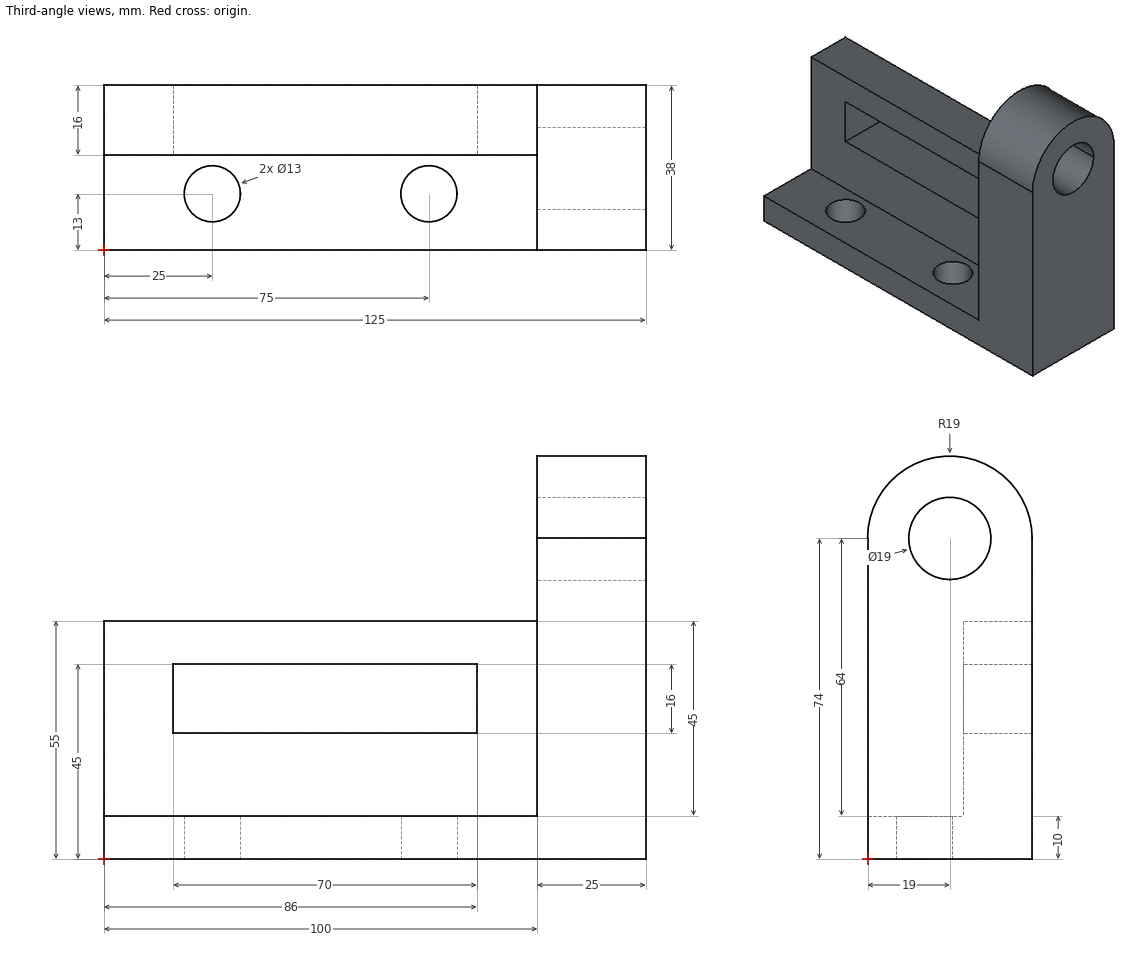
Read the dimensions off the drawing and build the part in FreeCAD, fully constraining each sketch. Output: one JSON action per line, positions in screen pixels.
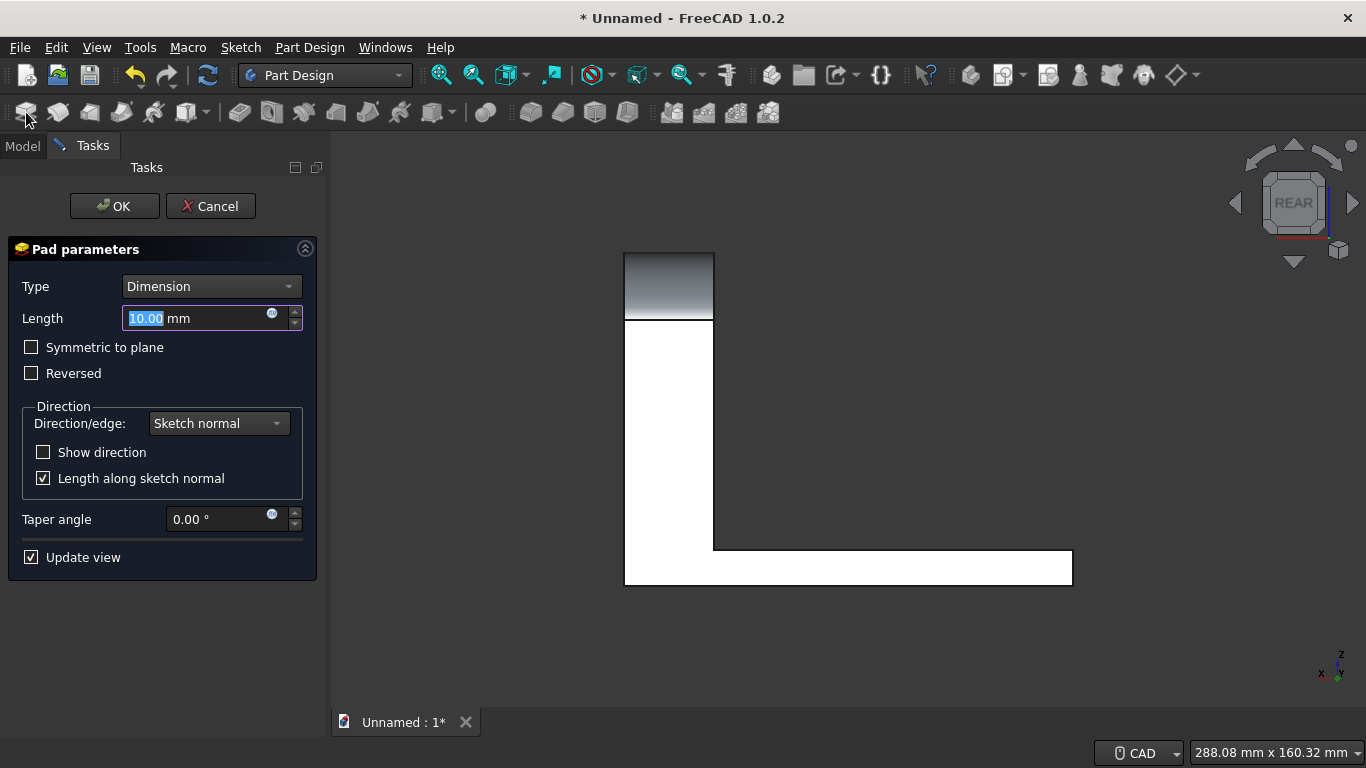
{"action": "type", "text": "16"}
{"action": "key", "text": "Tab"}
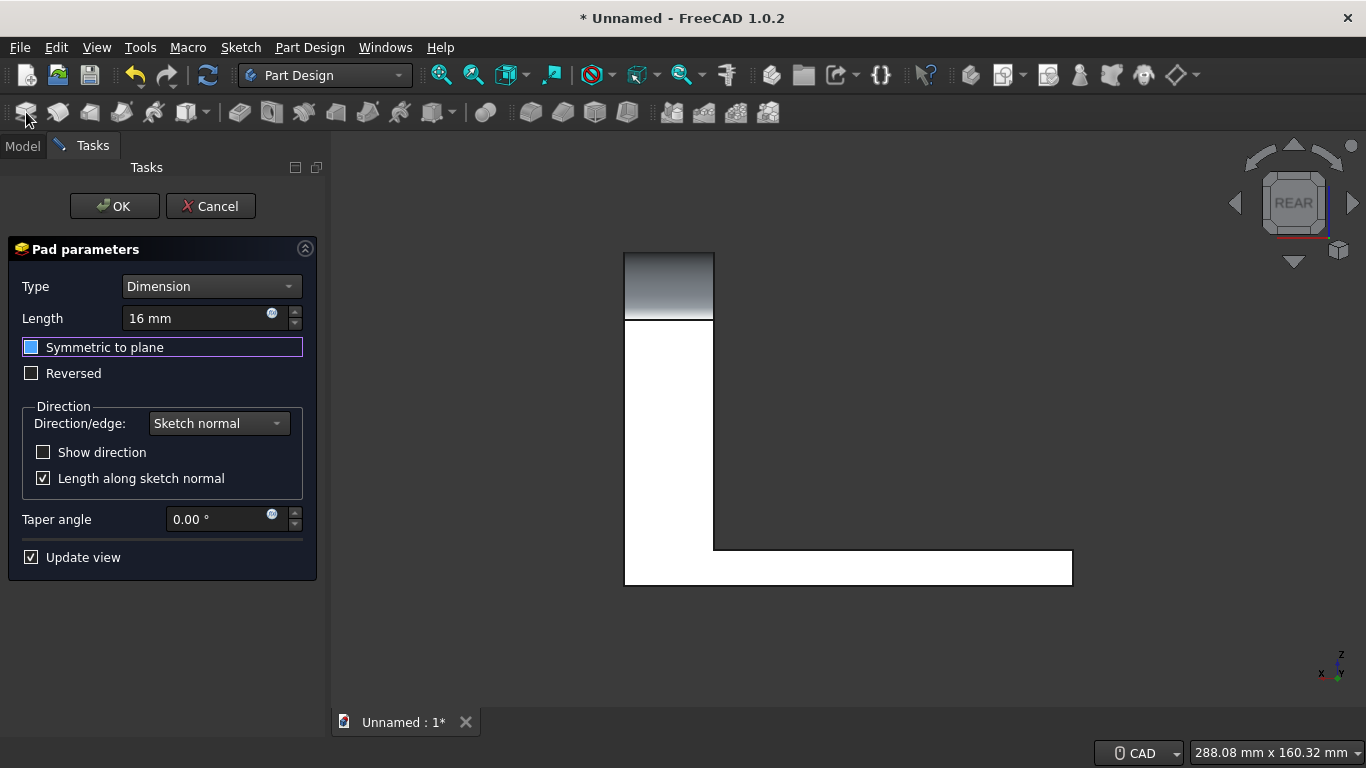
{"action": "left_click", "coordinate": [30, 373]}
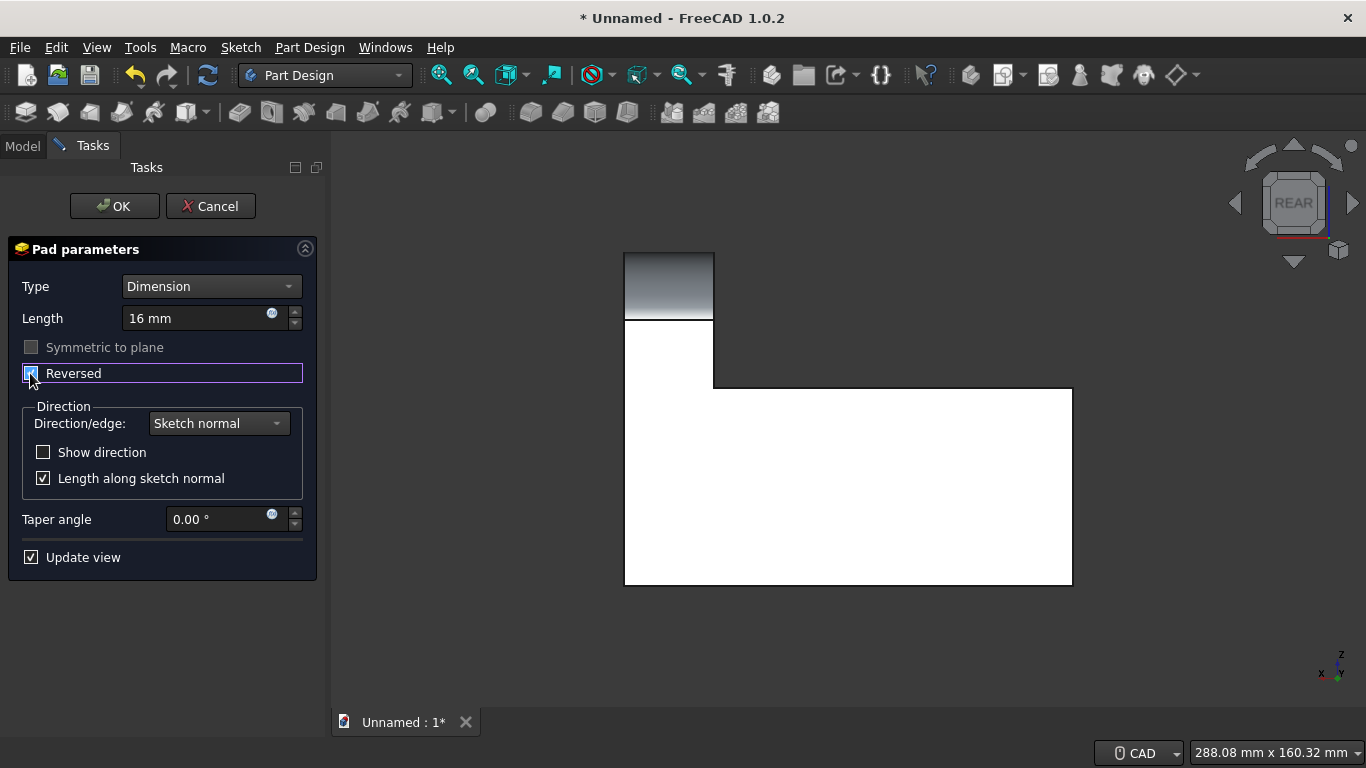
{"action": "left_click", "coordinate": [115, 206]}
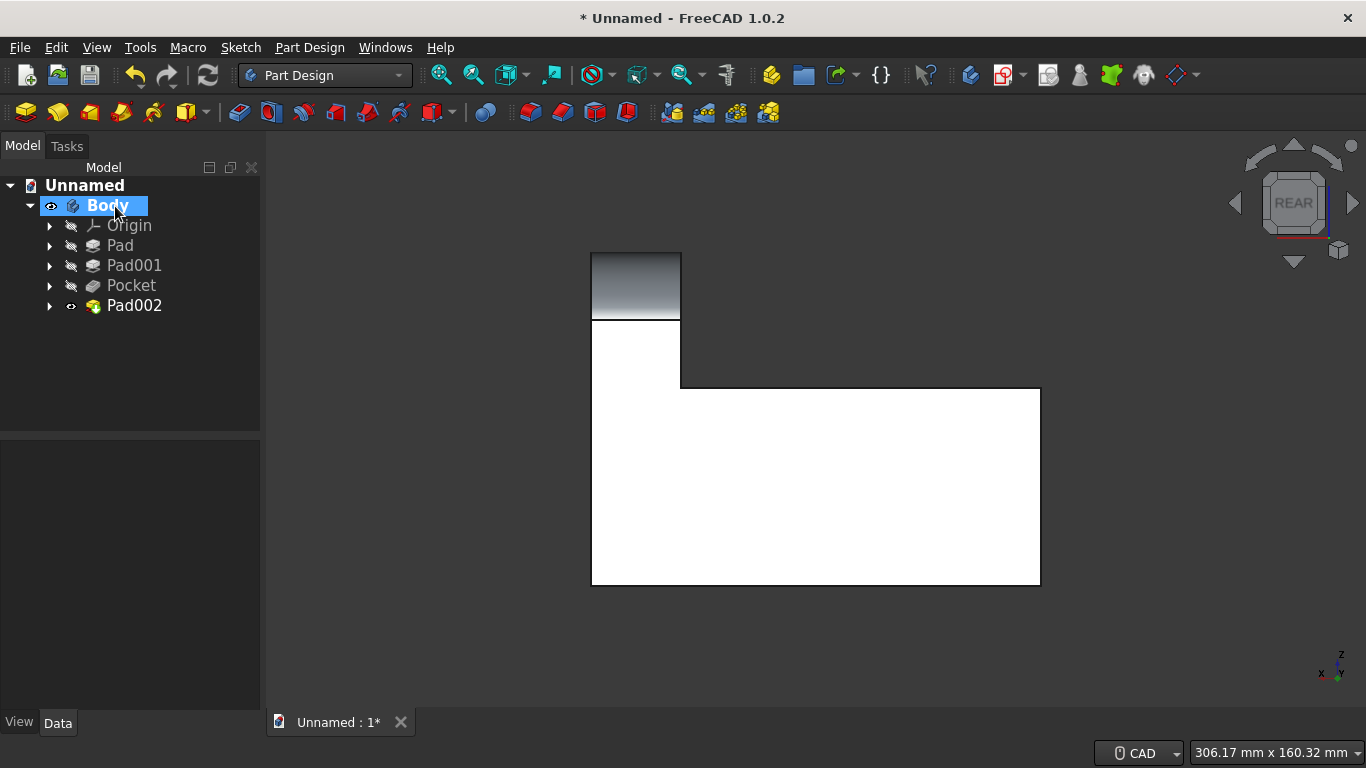
{"action": "left_click", "coordinate": [688, 490]}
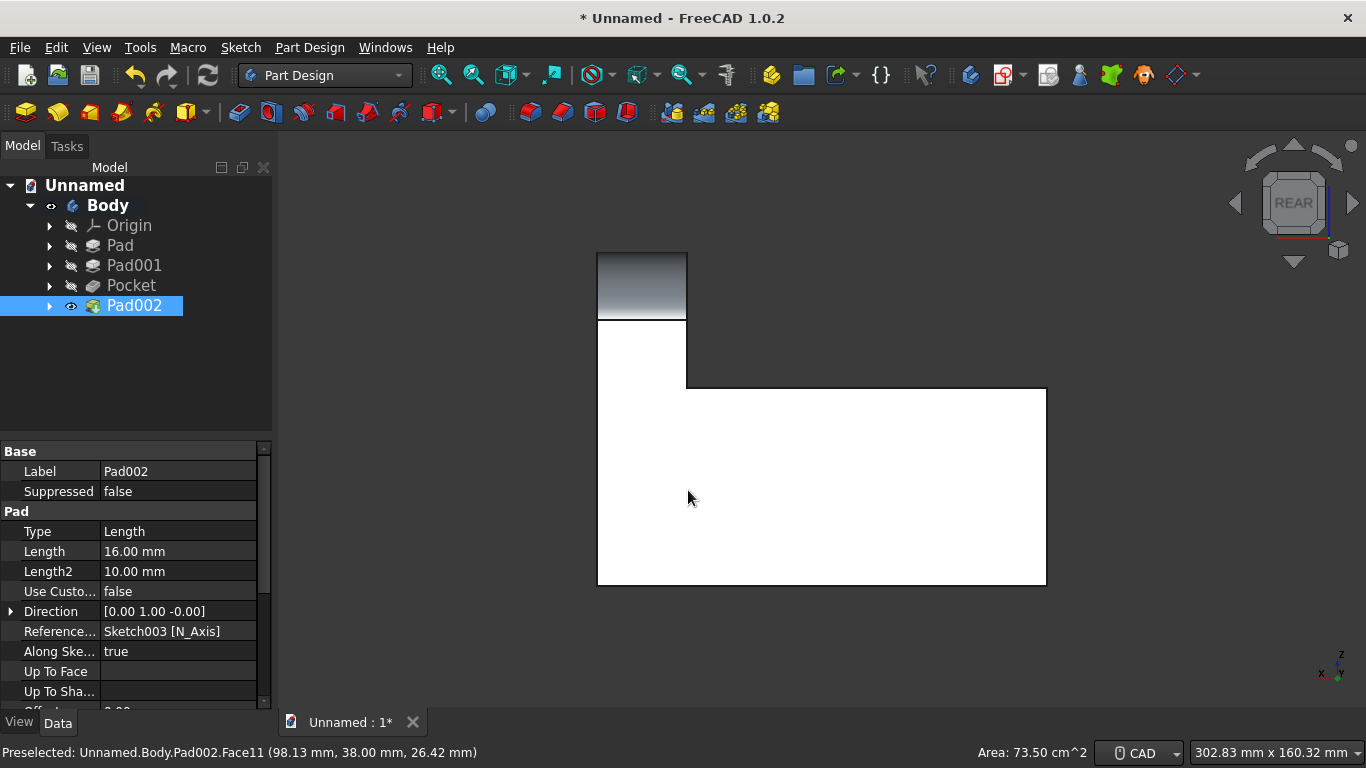
{"action": "left_click", "coordinate": [1004, 76]}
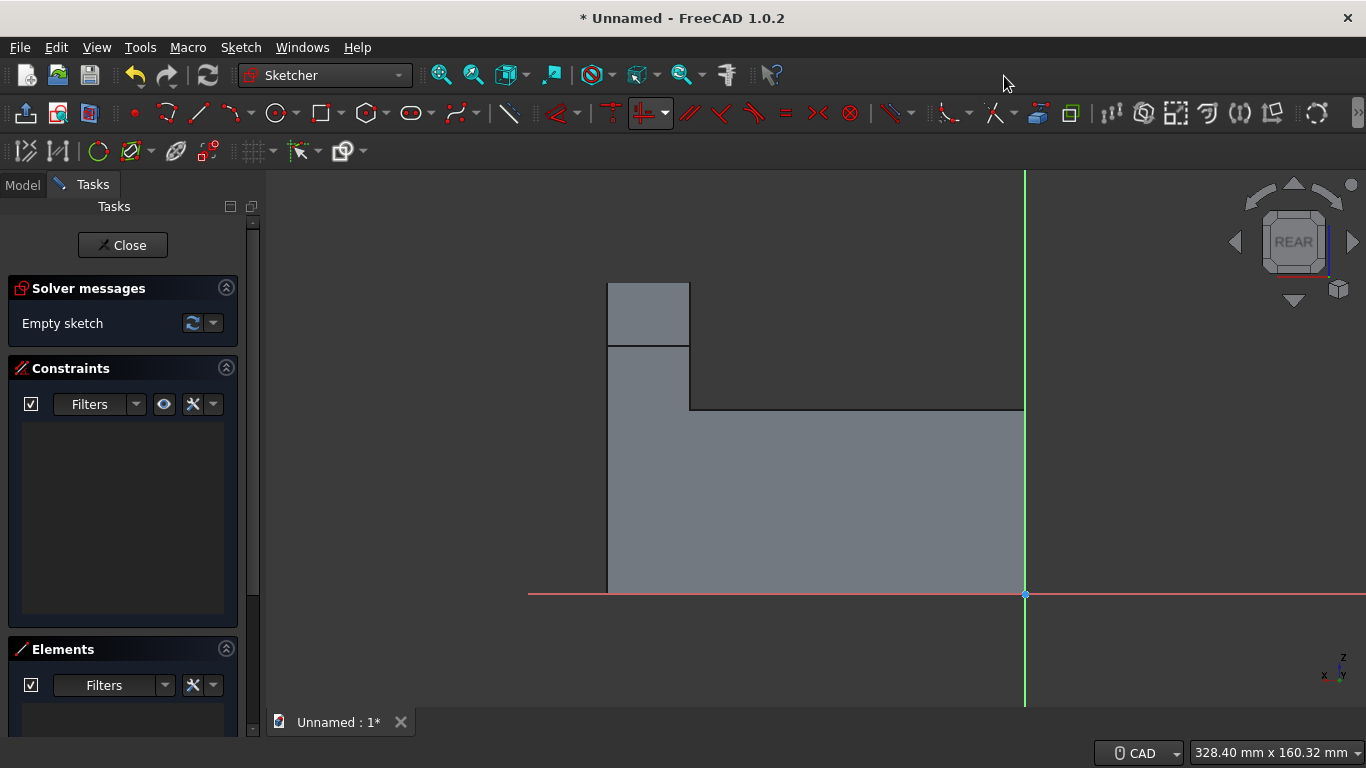
{"action": "scroll", "coordinate": [991, 584], "scroll_direction": "up", "scroll_amount": 4}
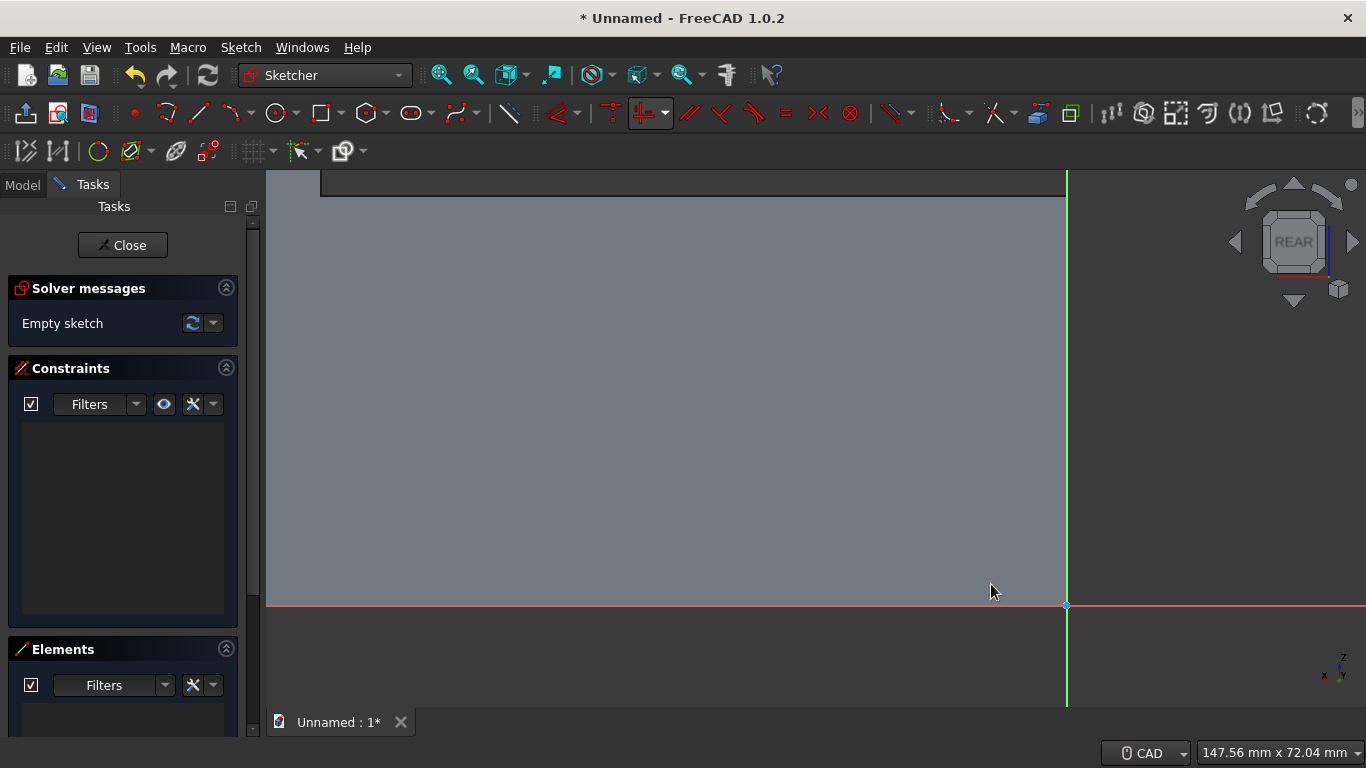
{"action": "left_click", "coordinate": [322, 114]}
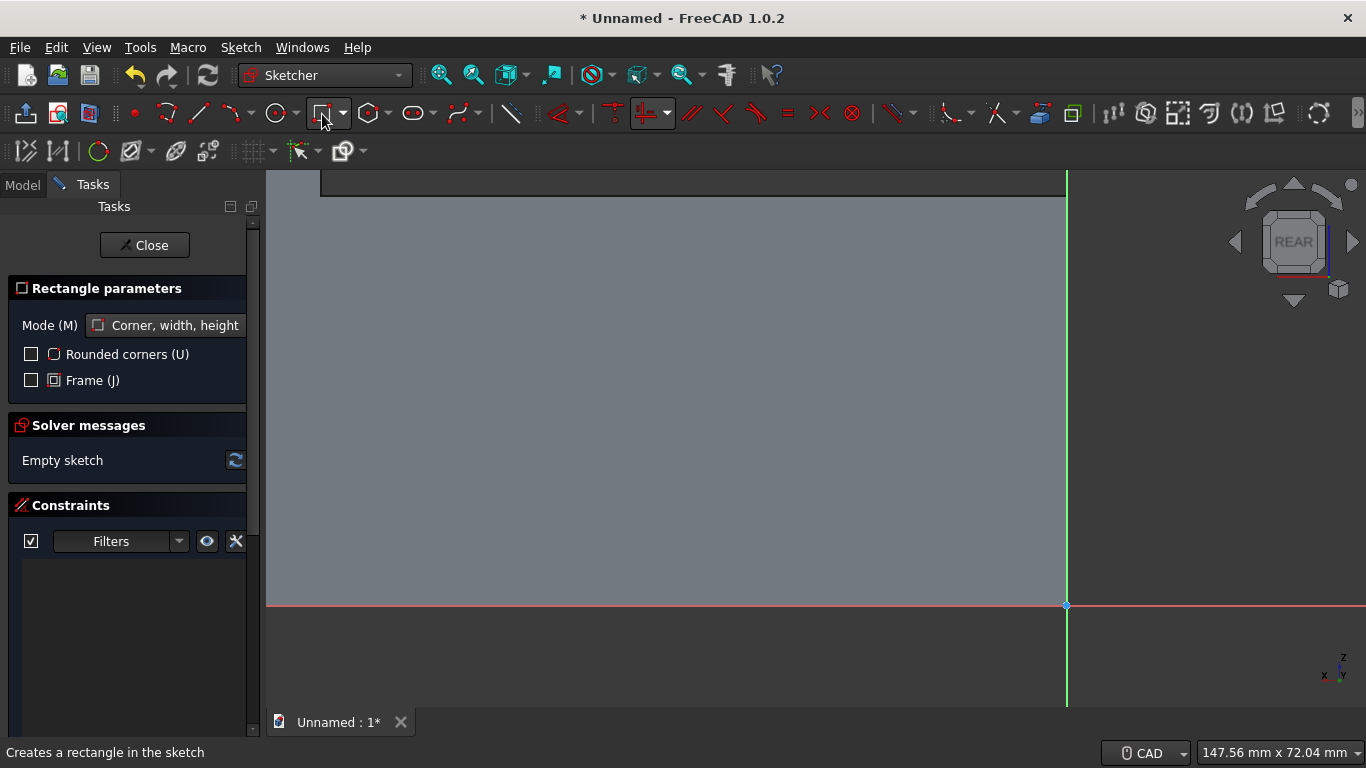
{"action": "left_click", "coordinate": [426, 270]}
{"action": "left_click", "coordinate": [947, 389]}
{"action": "key", "text": "Escape"}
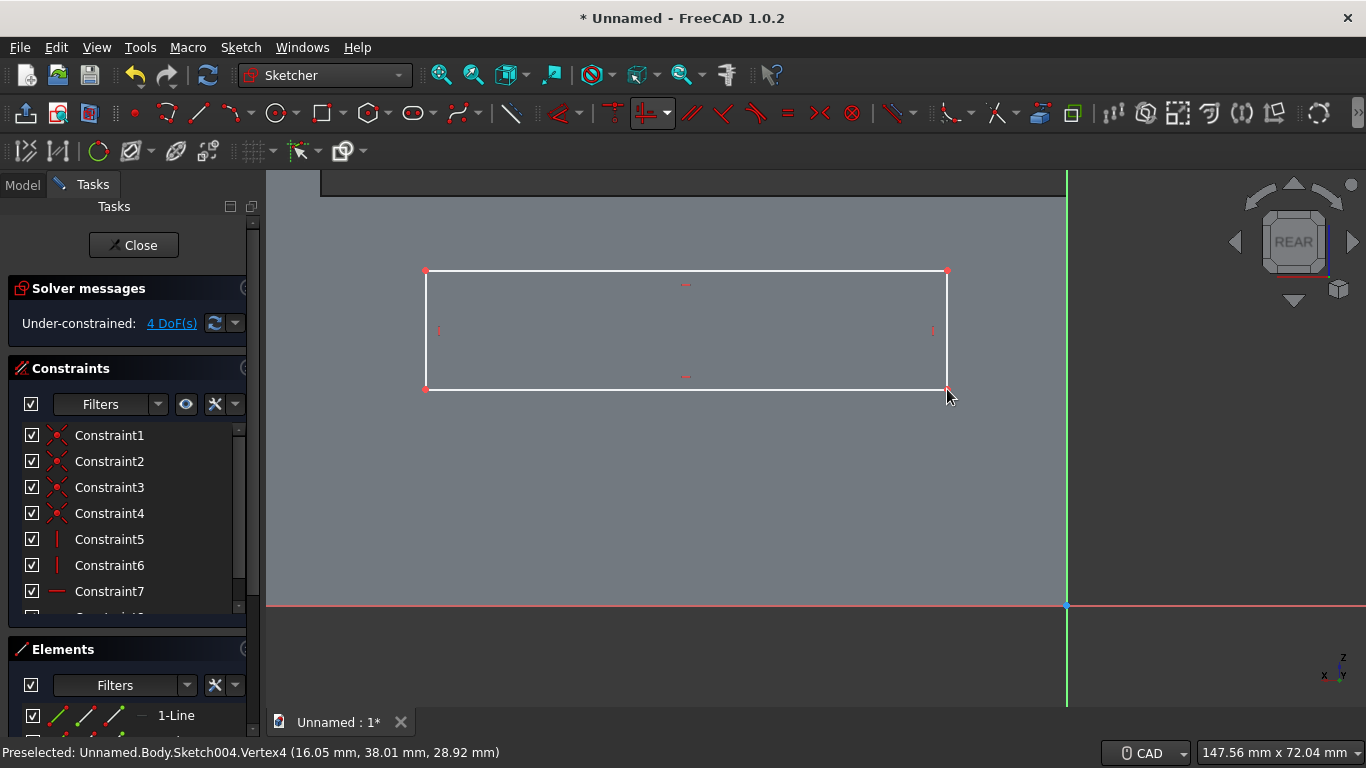
{"action": "left_click", "coordinate": [558, 114]}